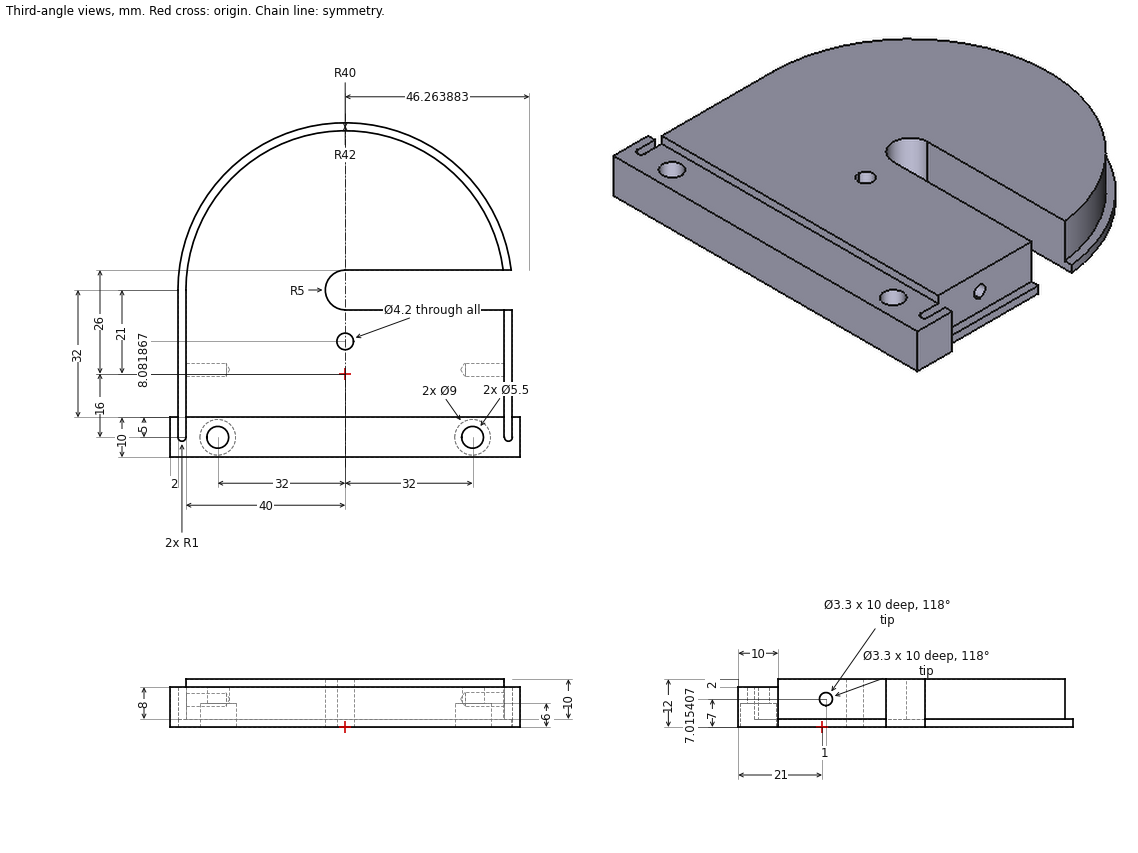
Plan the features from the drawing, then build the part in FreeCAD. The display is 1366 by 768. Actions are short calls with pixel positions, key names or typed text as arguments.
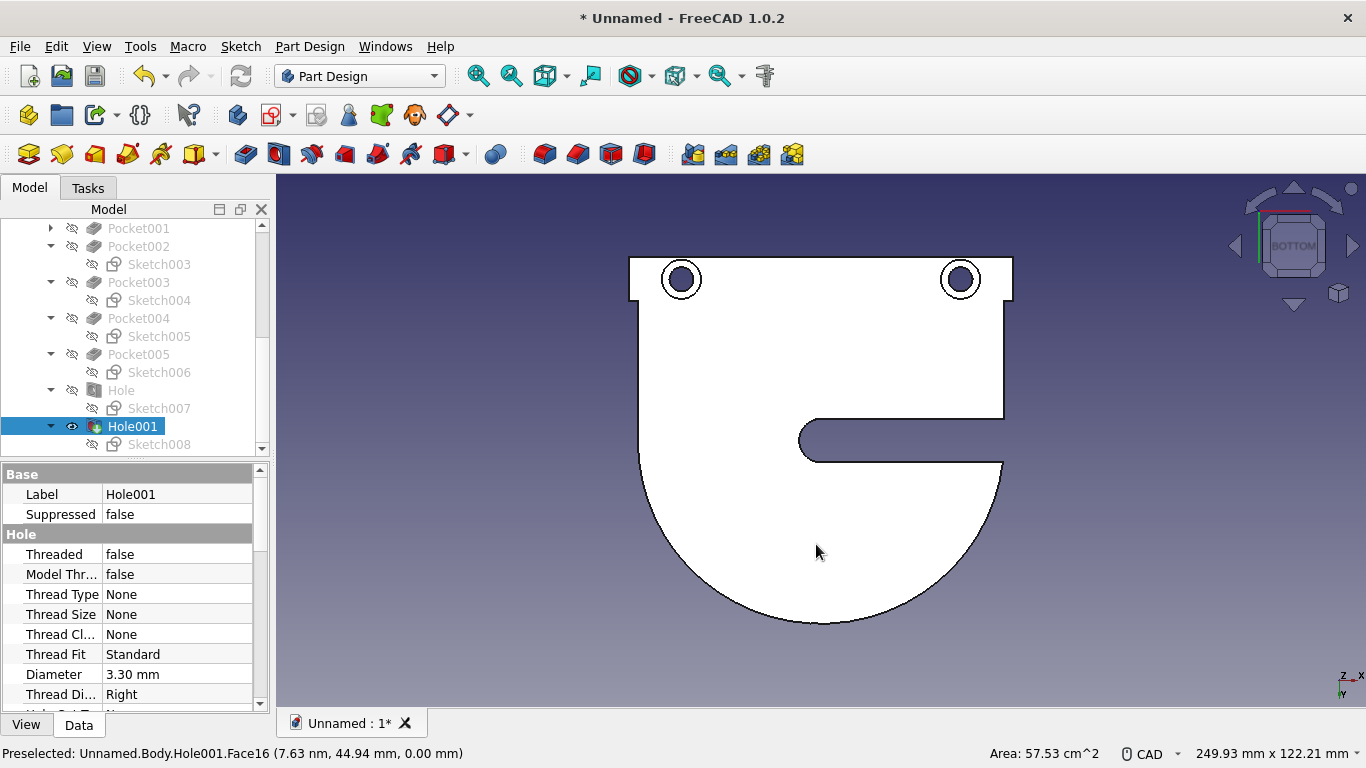
click(270, 116)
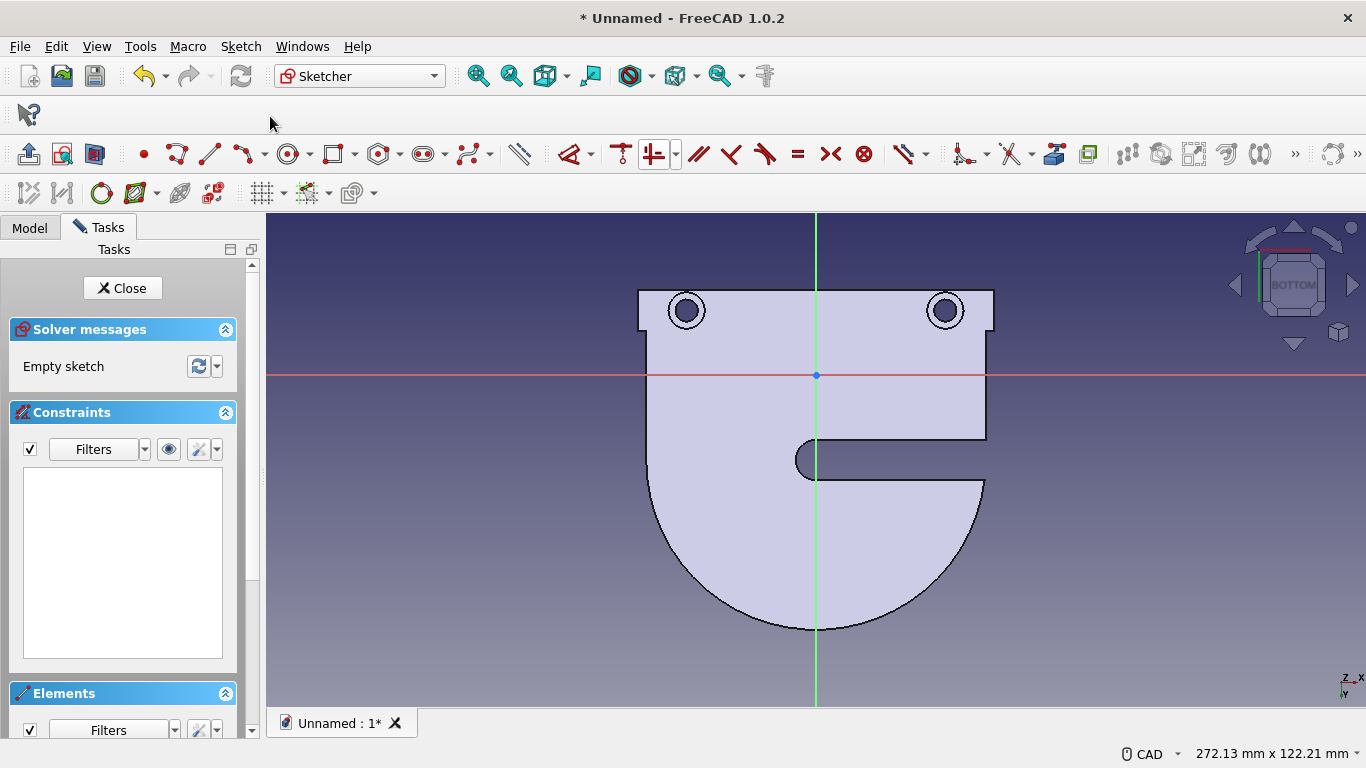
scroll(827, 386, up, 10)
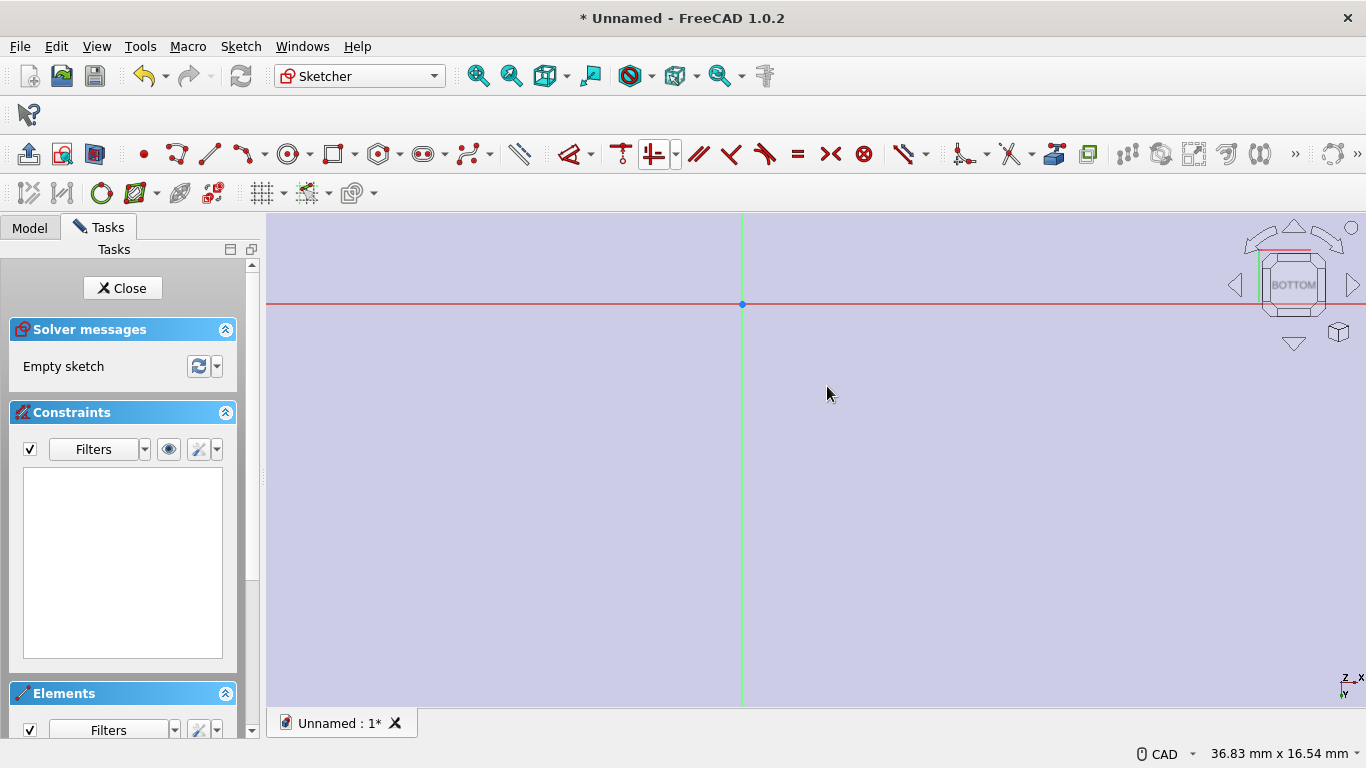
key(g)
key(c)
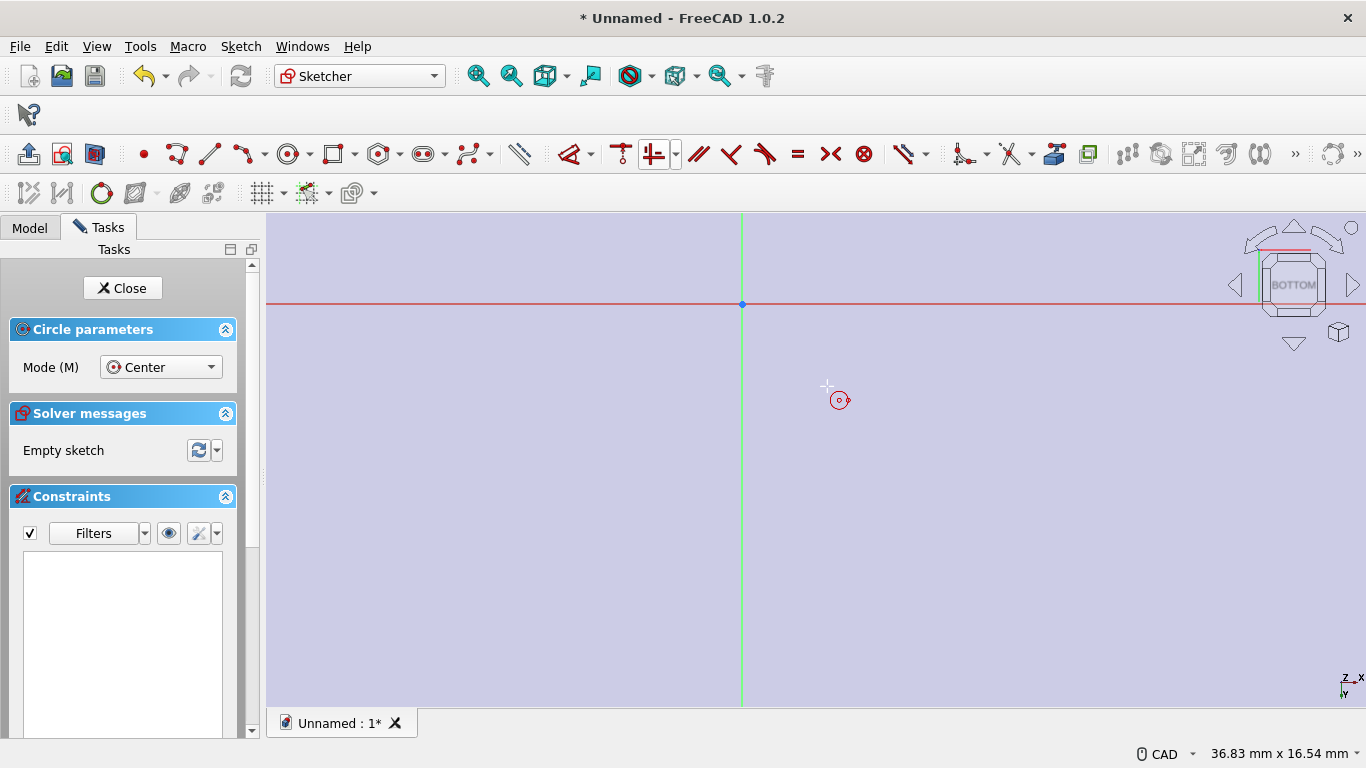
click(742, 545)
click(787, 501)
key(Escape)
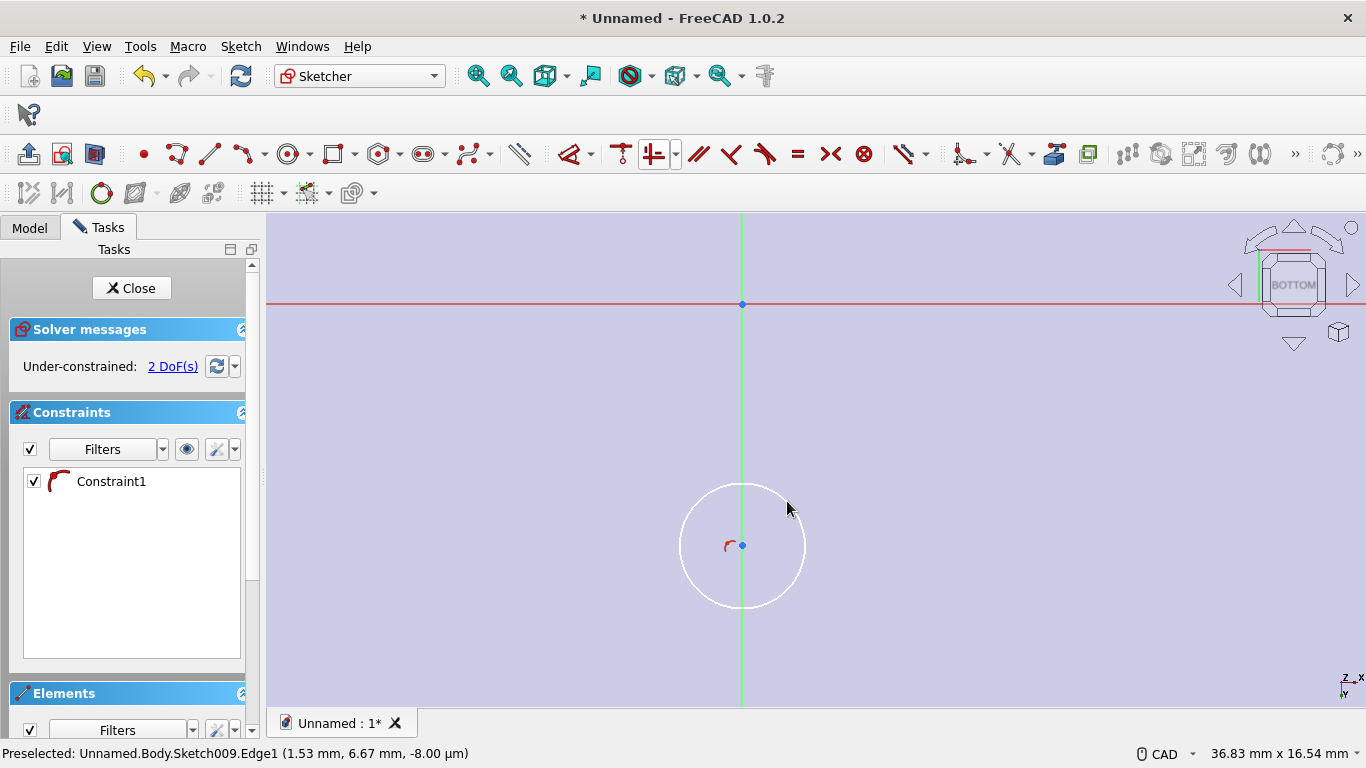
click(568, 154)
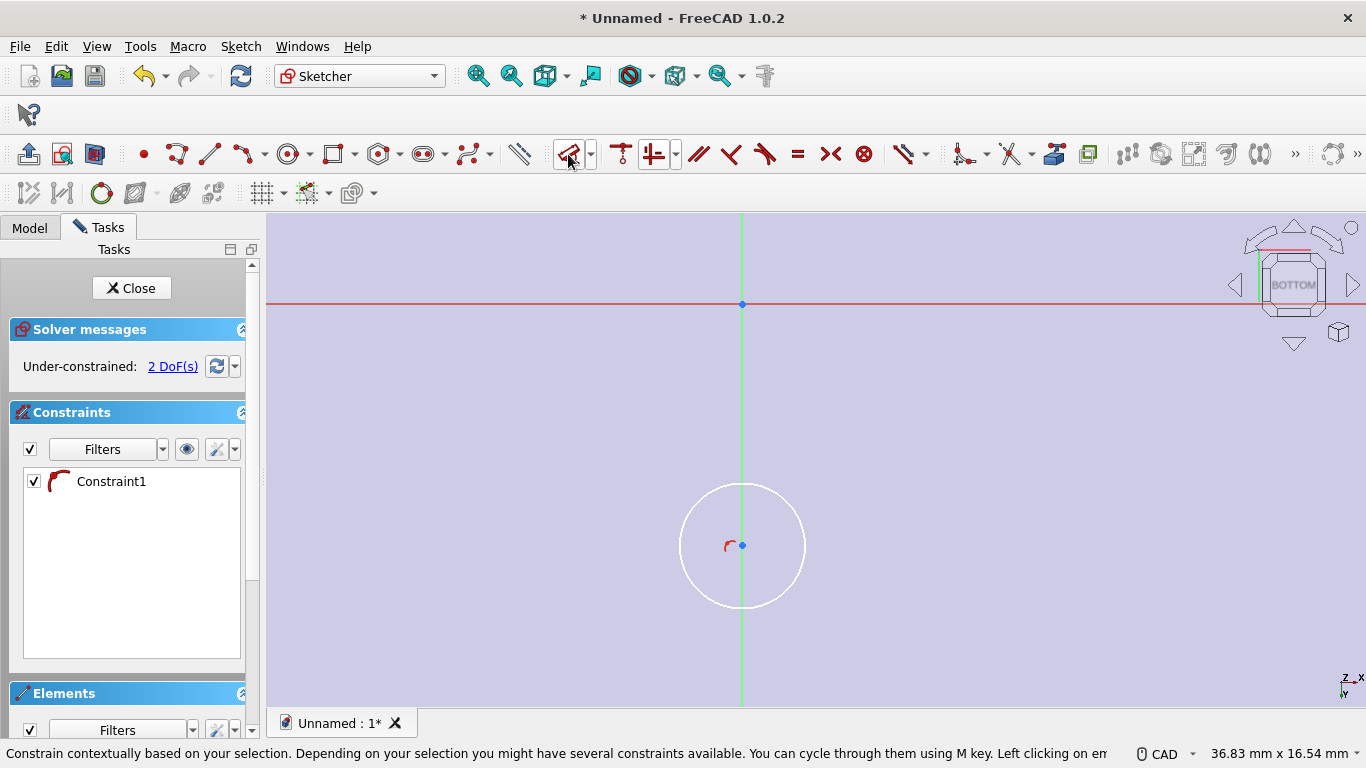
click(787, 502)
click(810, 480)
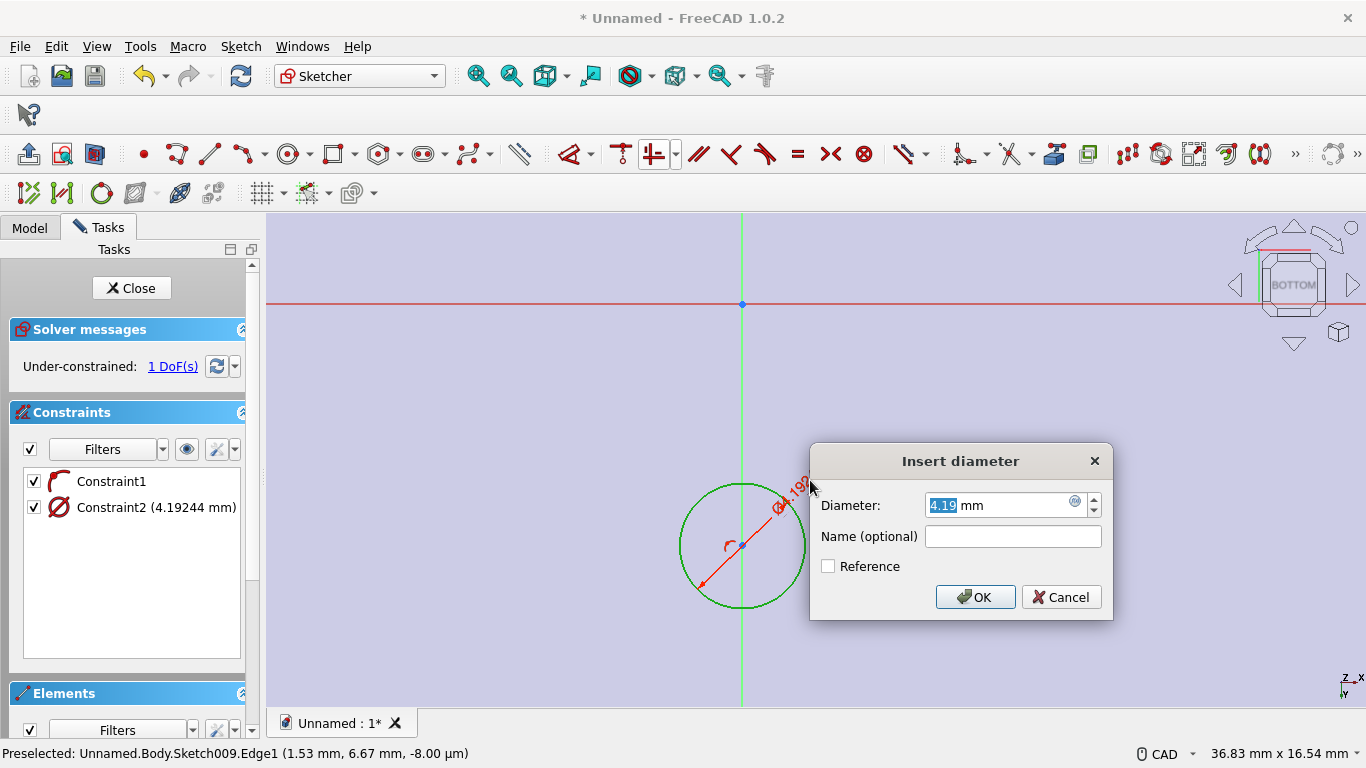
text(4.2)
key(Return)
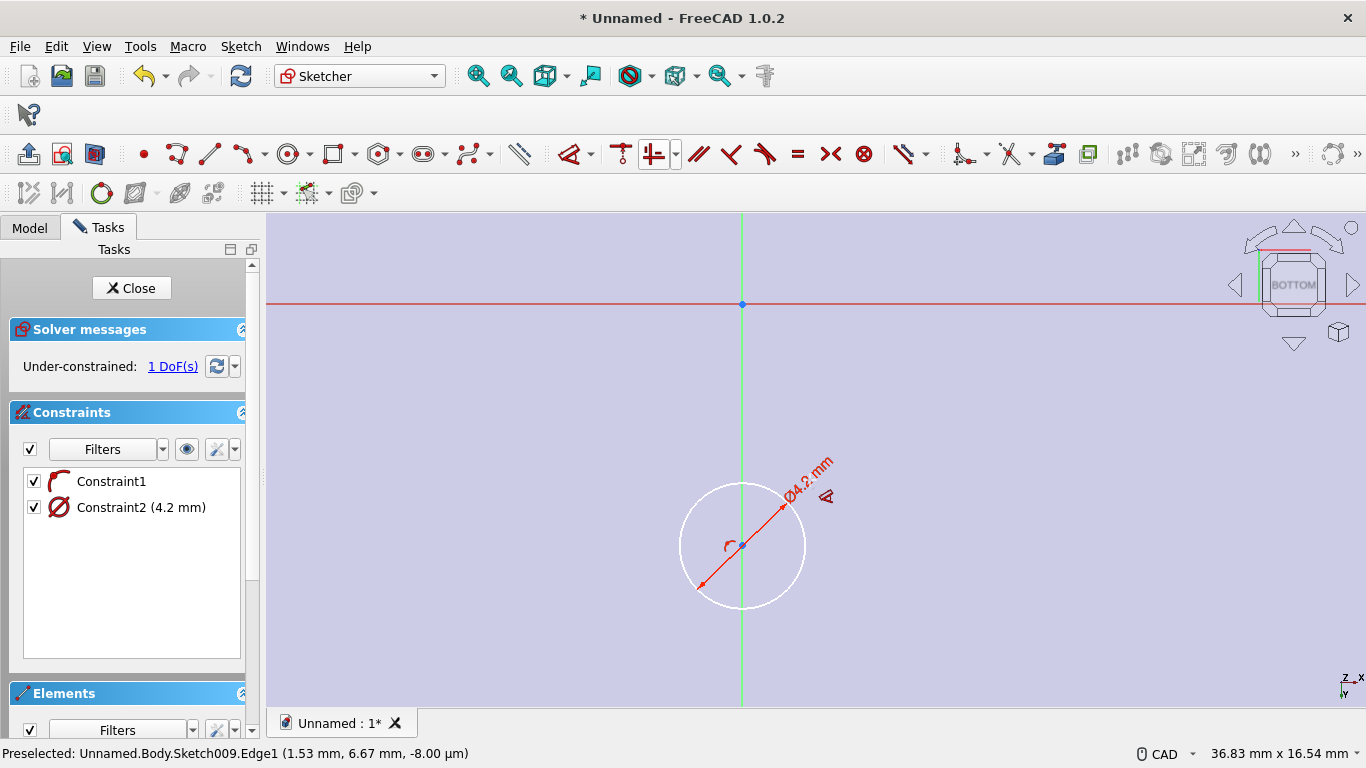
click(742, 546)
click(776, 425)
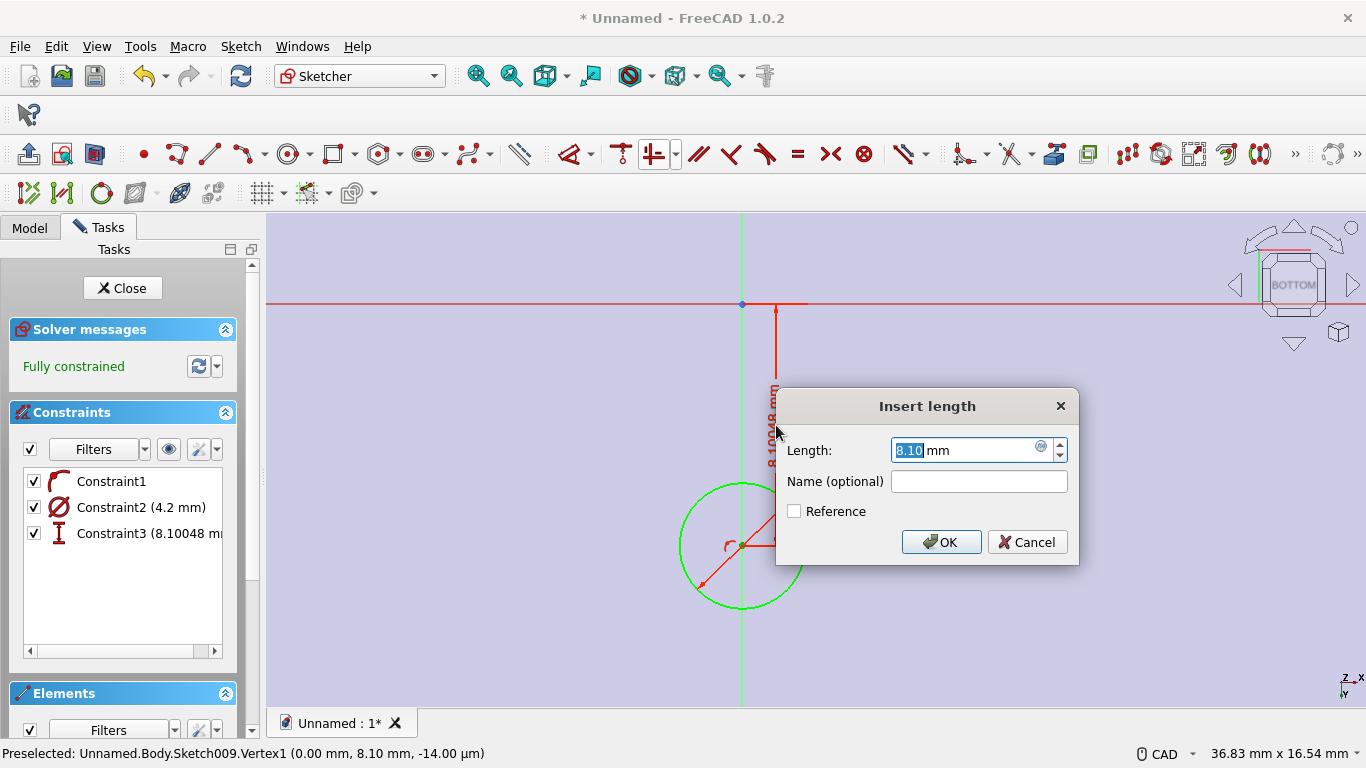
text(8.081867)
key(Return)
key(Escape)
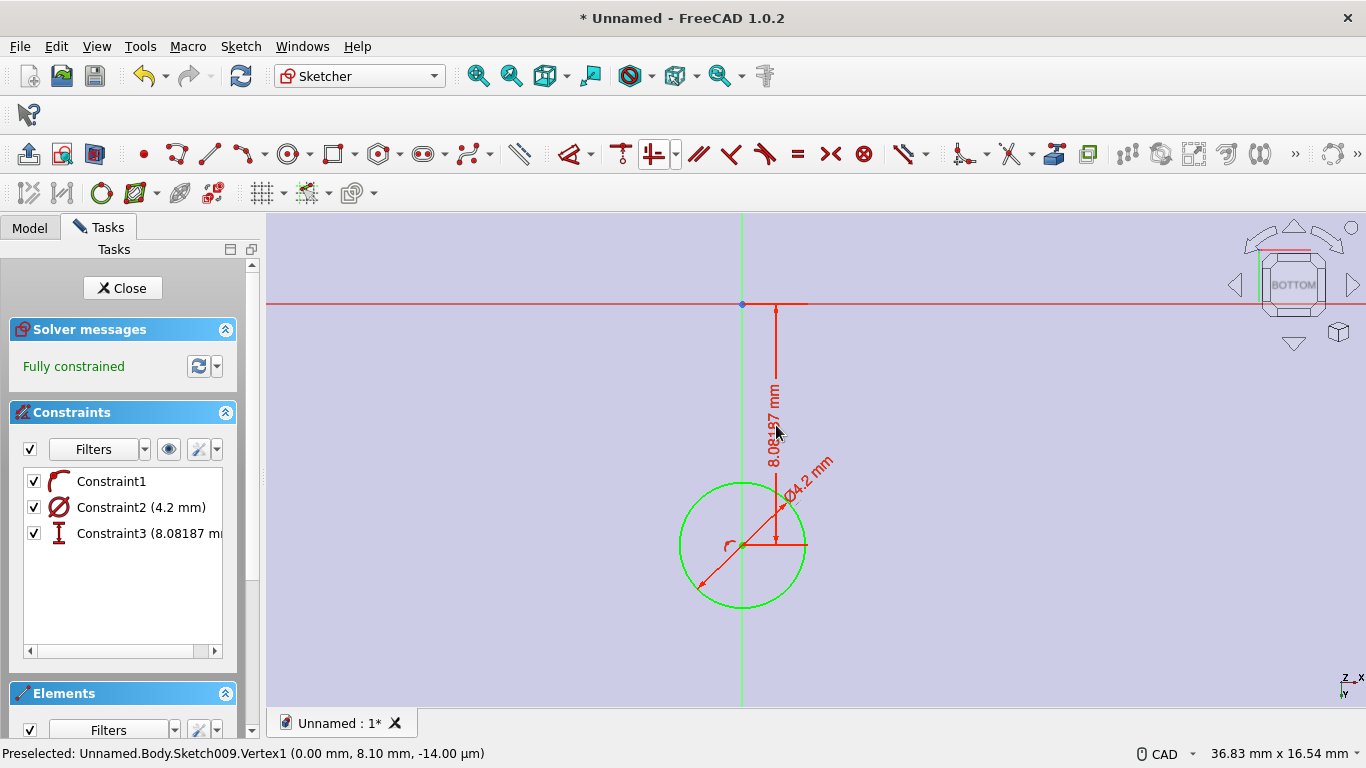
click(123, 288)